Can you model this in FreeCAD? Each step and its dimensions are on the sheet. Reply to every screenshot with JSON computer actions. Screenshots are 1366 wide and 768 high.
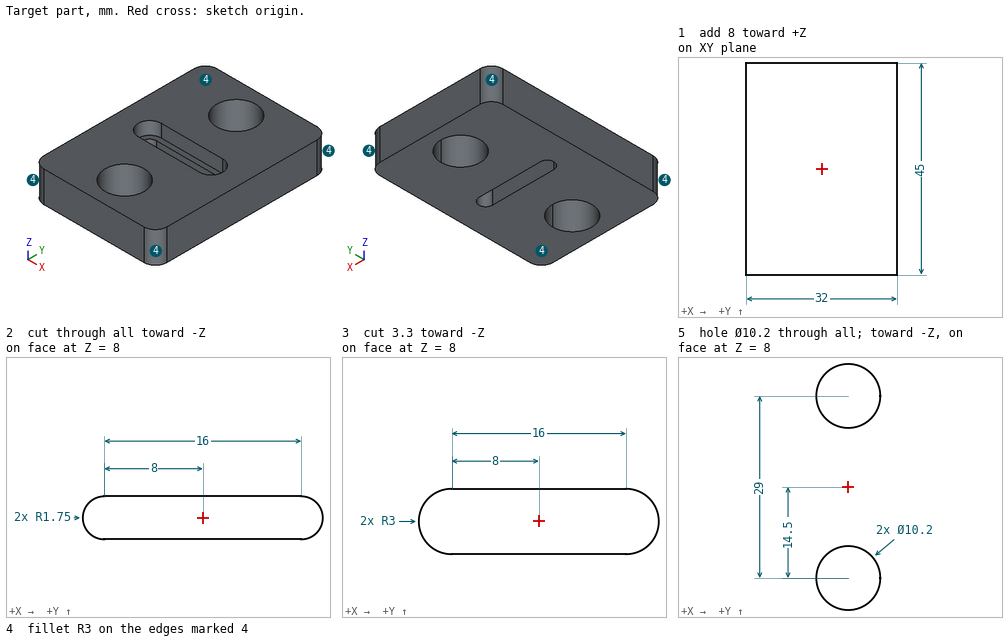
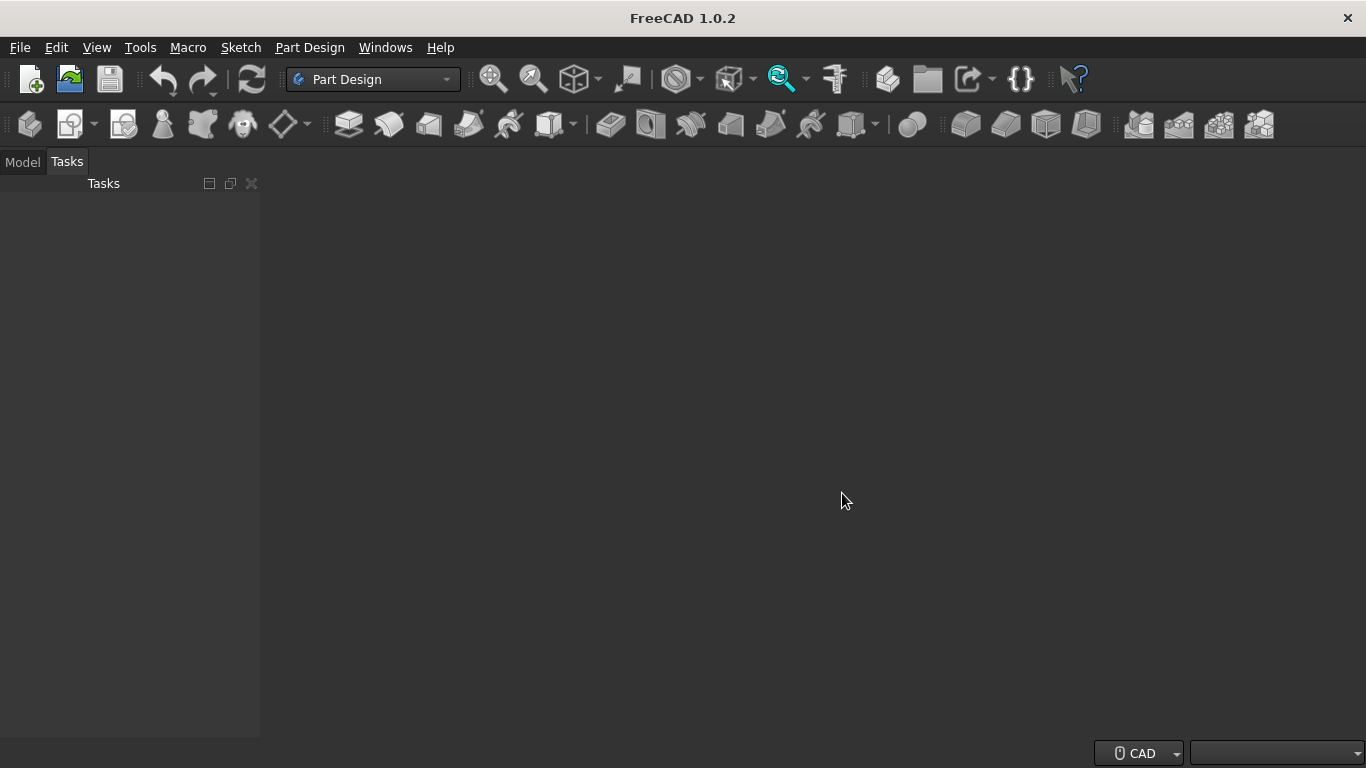
{"action": "key", "text": "ctrl+n"}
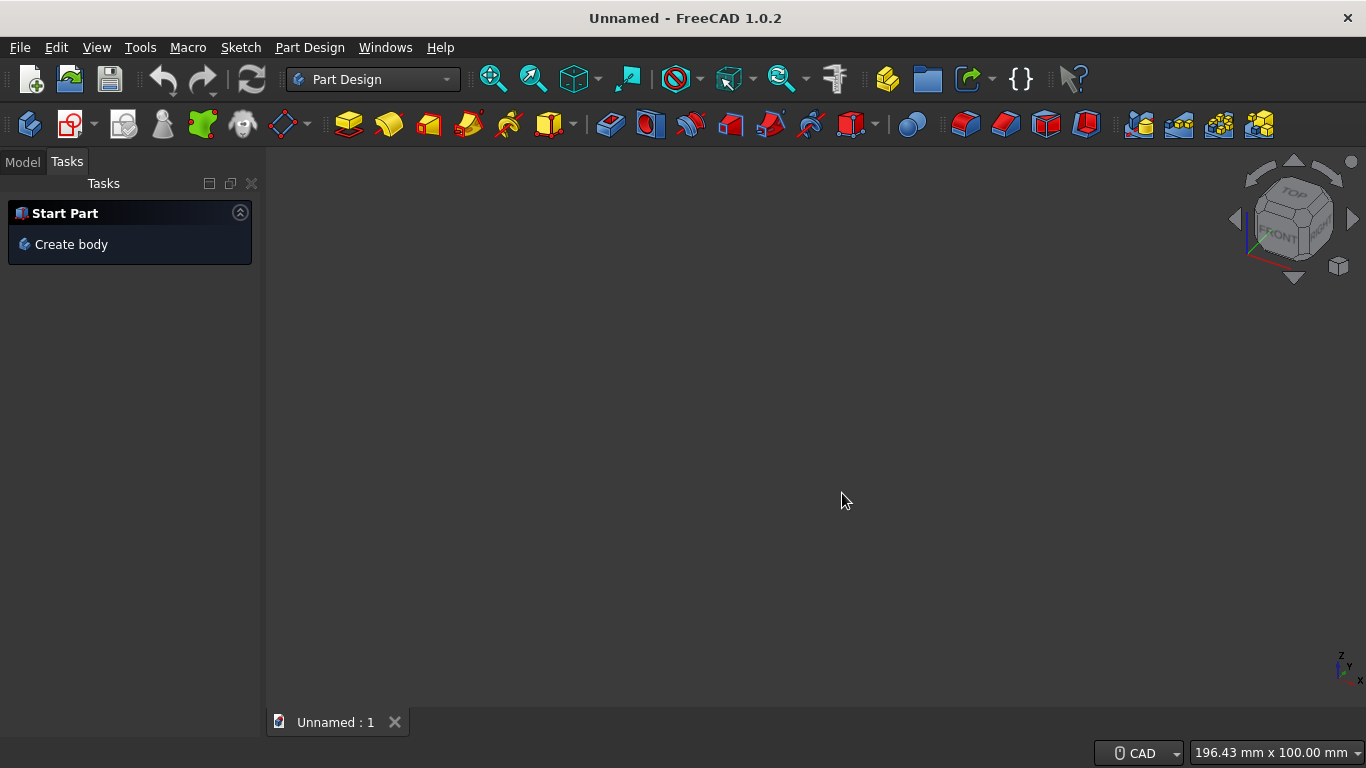
{"action": "left_click", "coordinate": [70, 124]}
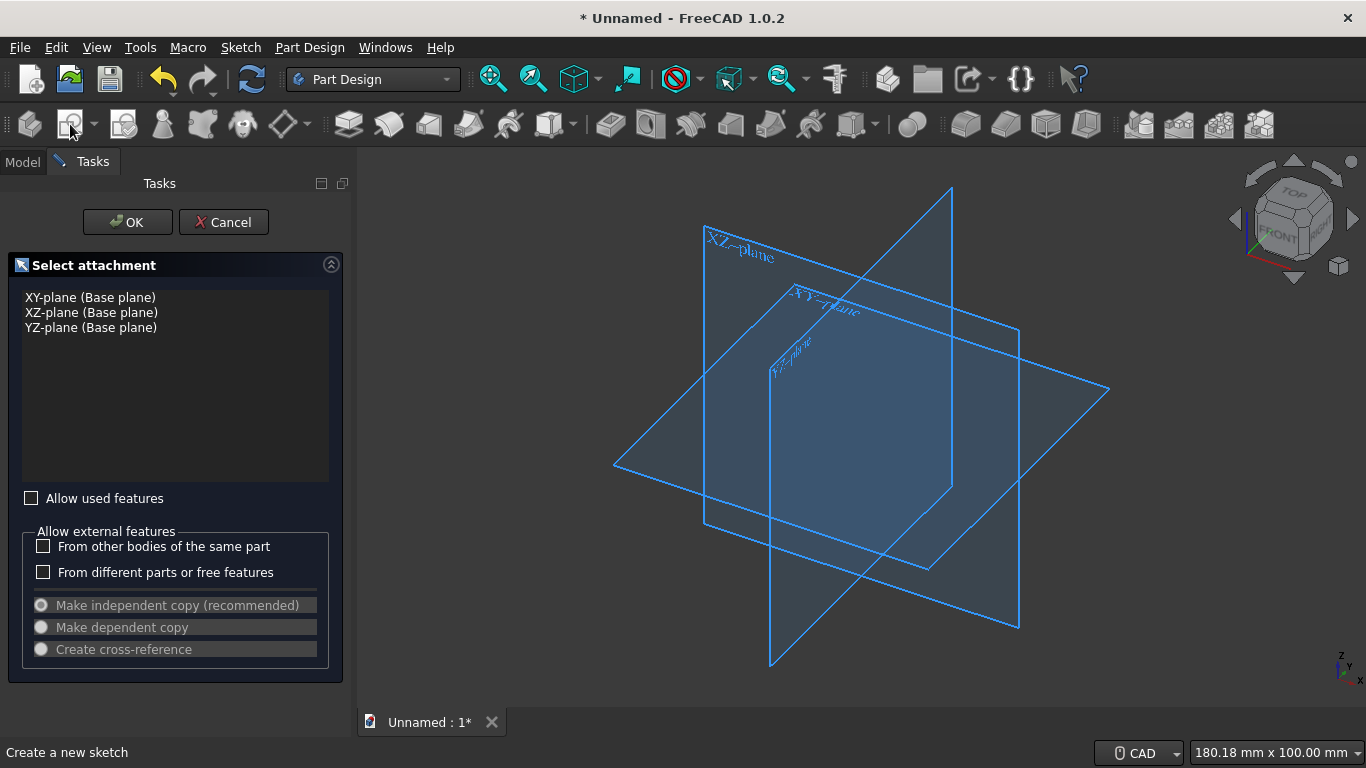
{"action": "left_click", "coordinate": [82, 298]}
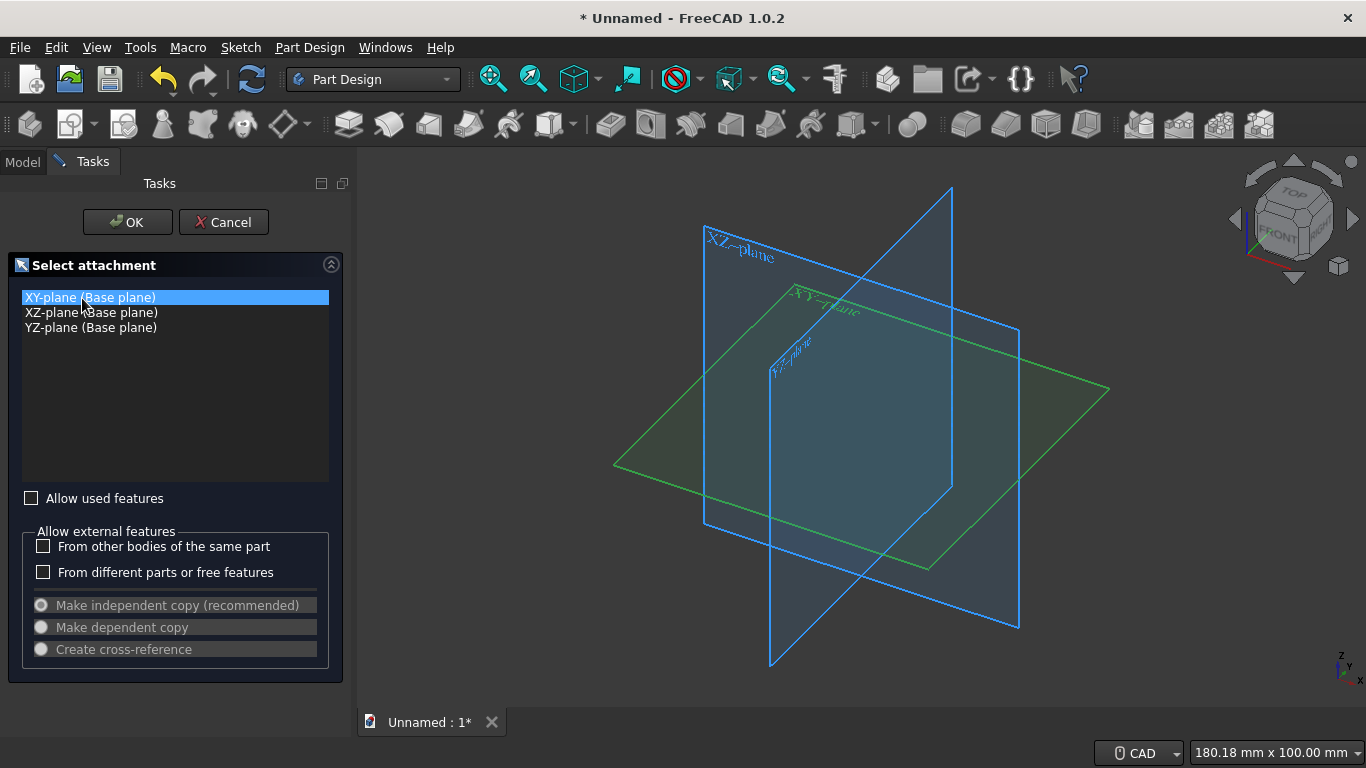
{"action": "left_click", "coordinate": [128, 222]}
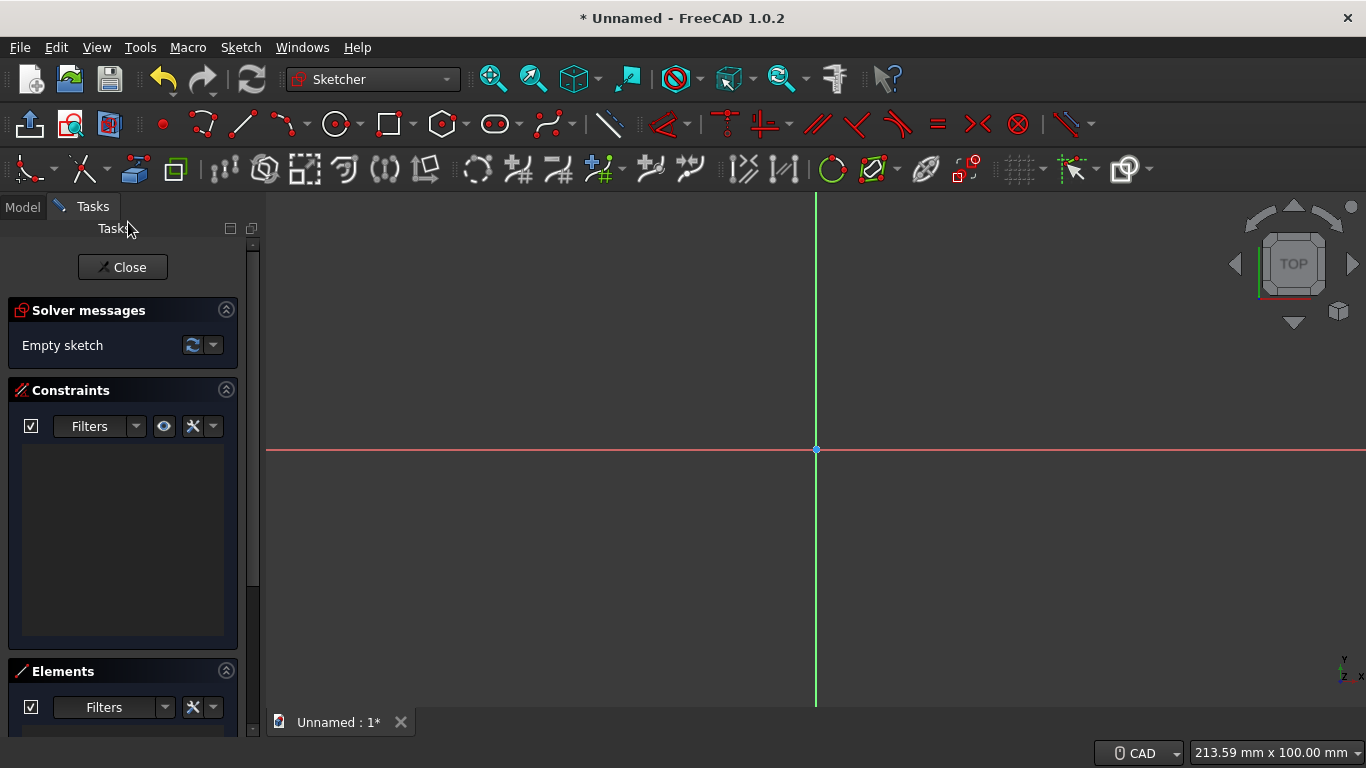
{"action": "scroll", "coordinate": [955, 450], "scroll_direction": "up", "scroll_amount": 2}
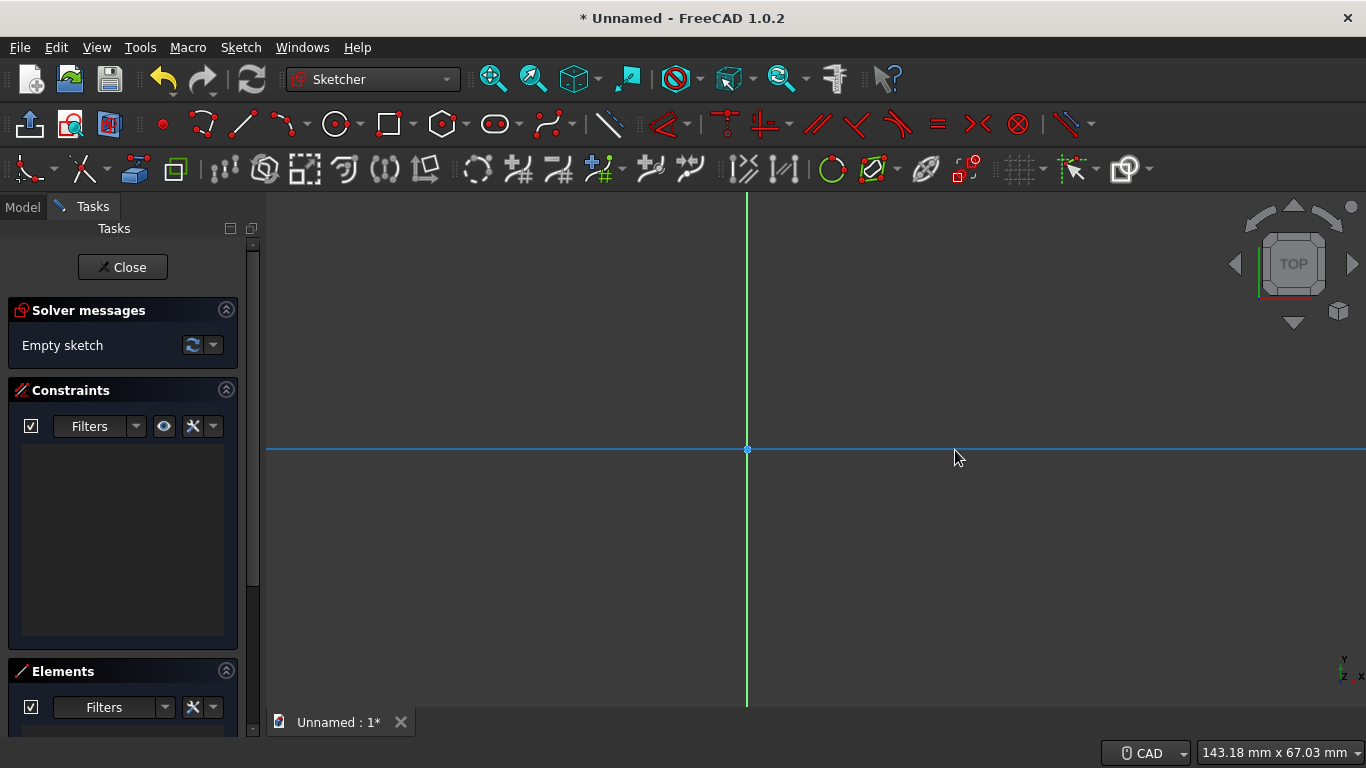
{"action": "key", "text": "g v"}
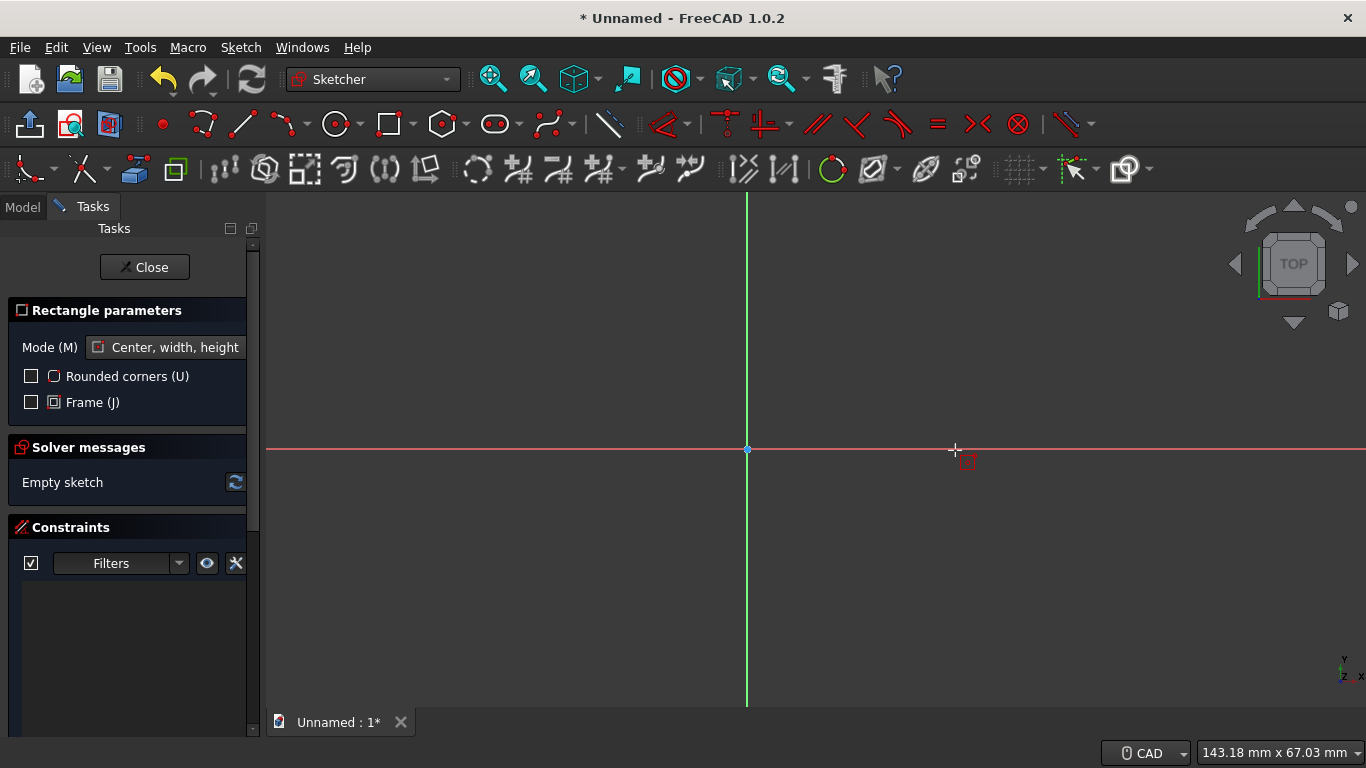
{"action": "left_click", "coordinate": [747, 449]}
{"action": "mouse_move", "coordinate": [870, 276]}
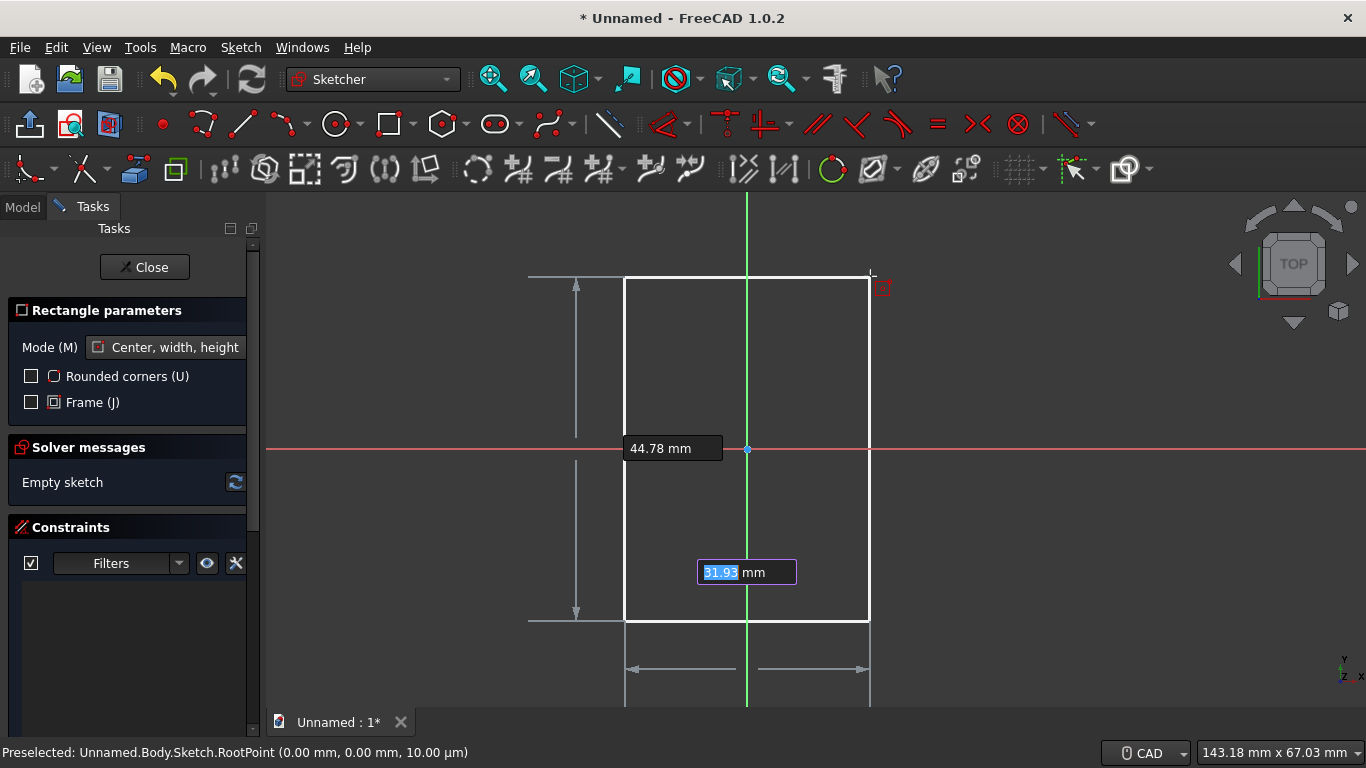
{"action": "type", "text": "32"}
{"action": "key", "text": "Tab"}
{"action": "type", "text": "45"}
{"action": "key", "text": "Return"}
{"action": "key", "text": "Escape"}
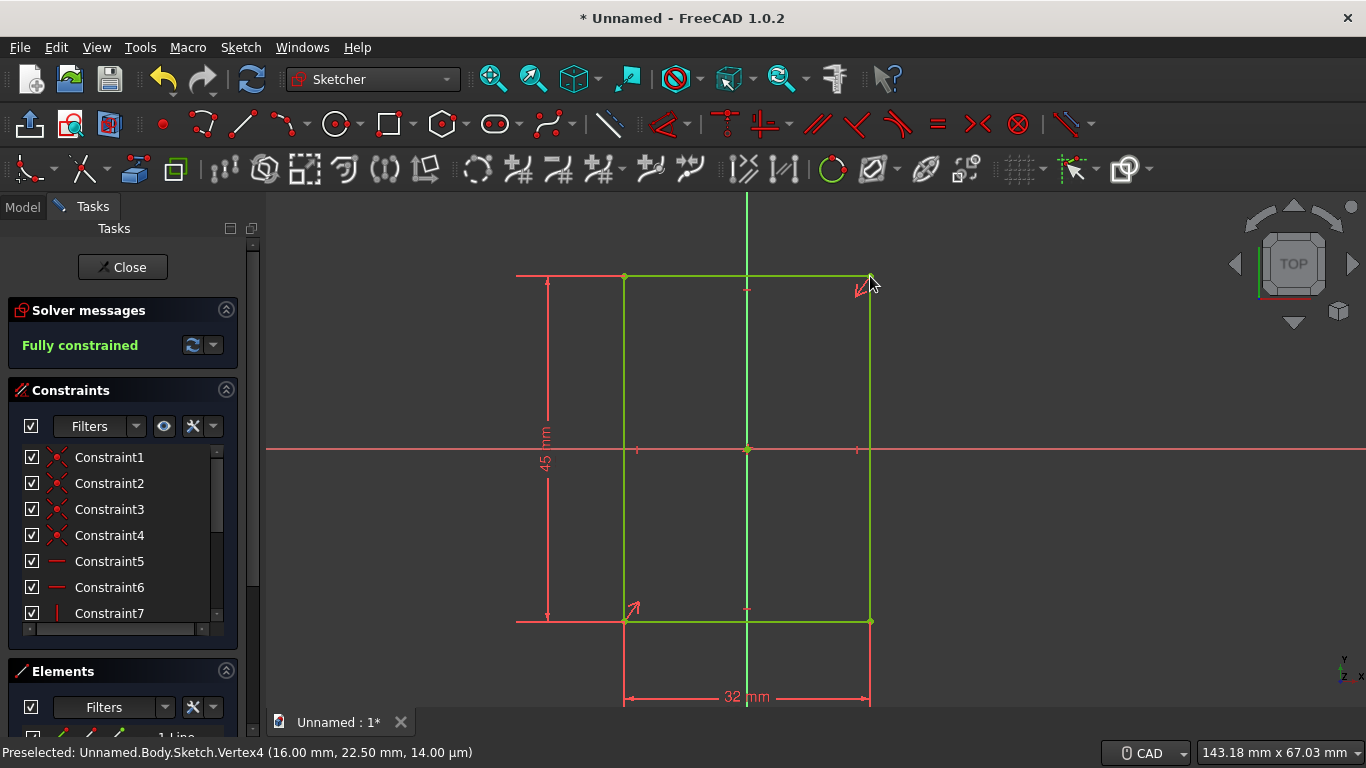
{"action": "left_click", "coordinate": [123, 267]}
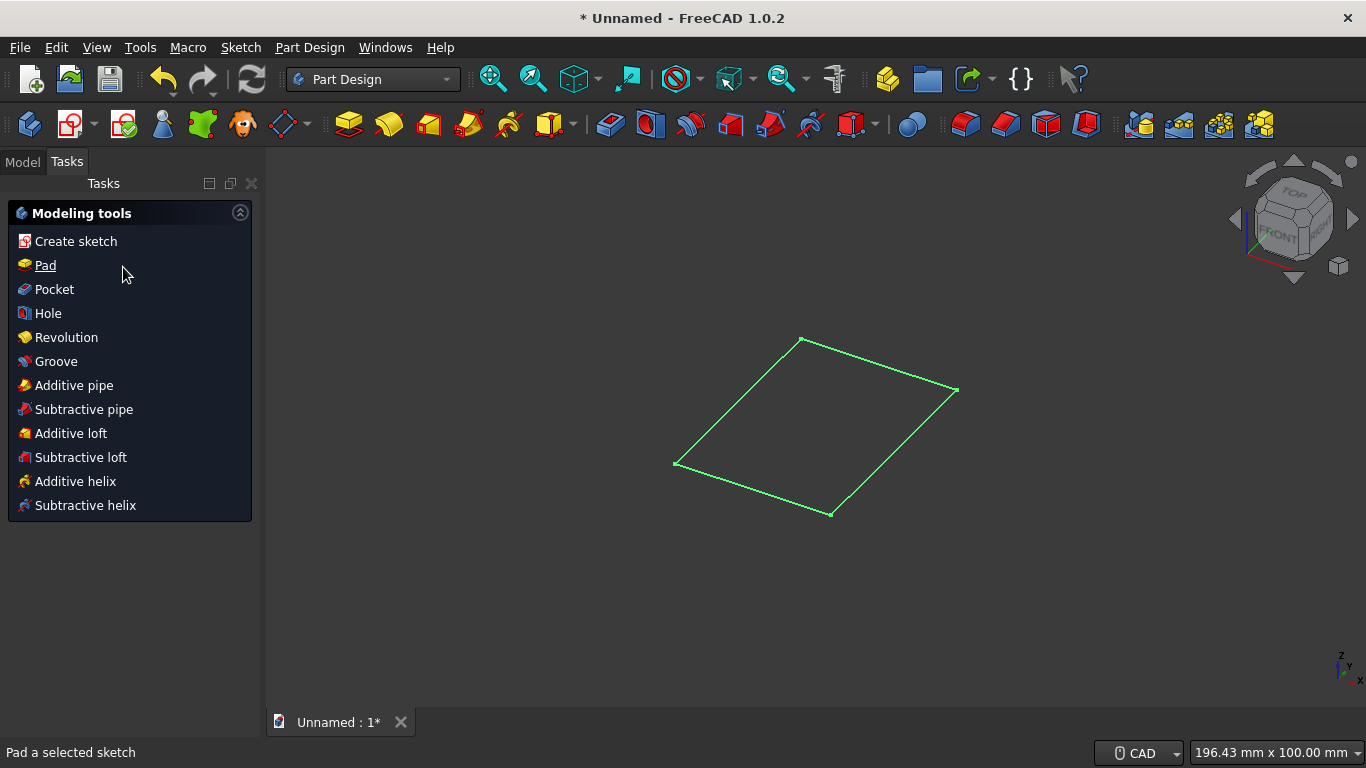
{"action": "left_click", "coordinate": [350, 124]}